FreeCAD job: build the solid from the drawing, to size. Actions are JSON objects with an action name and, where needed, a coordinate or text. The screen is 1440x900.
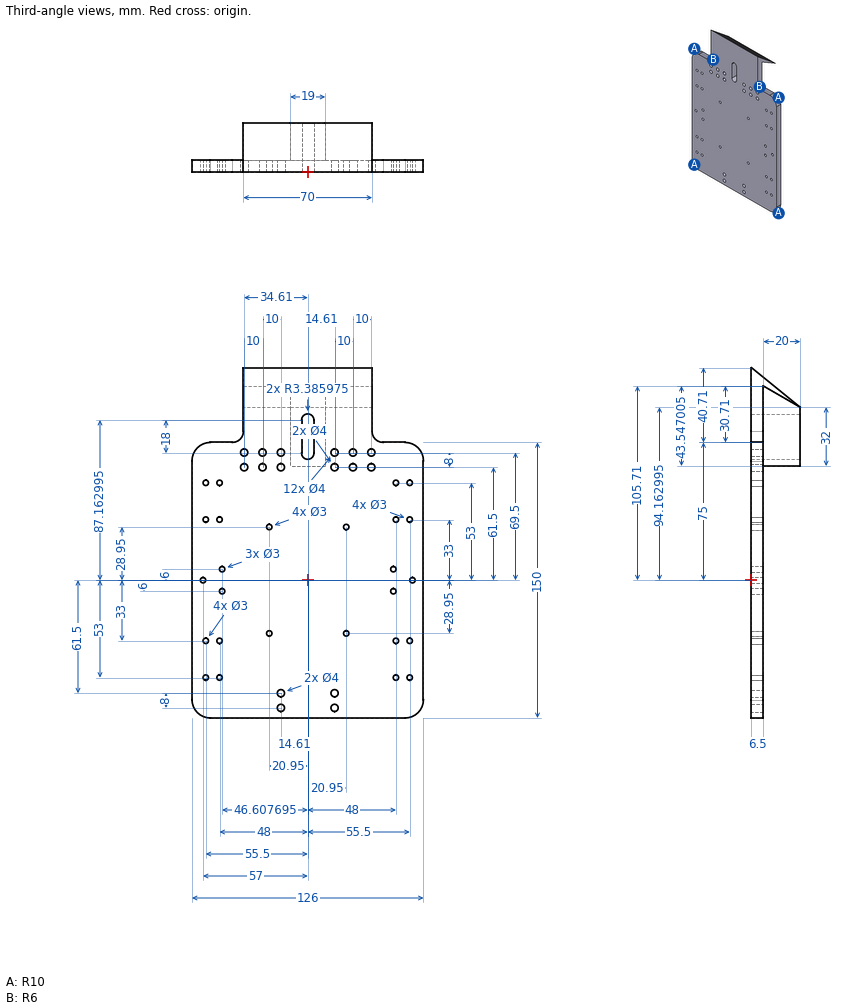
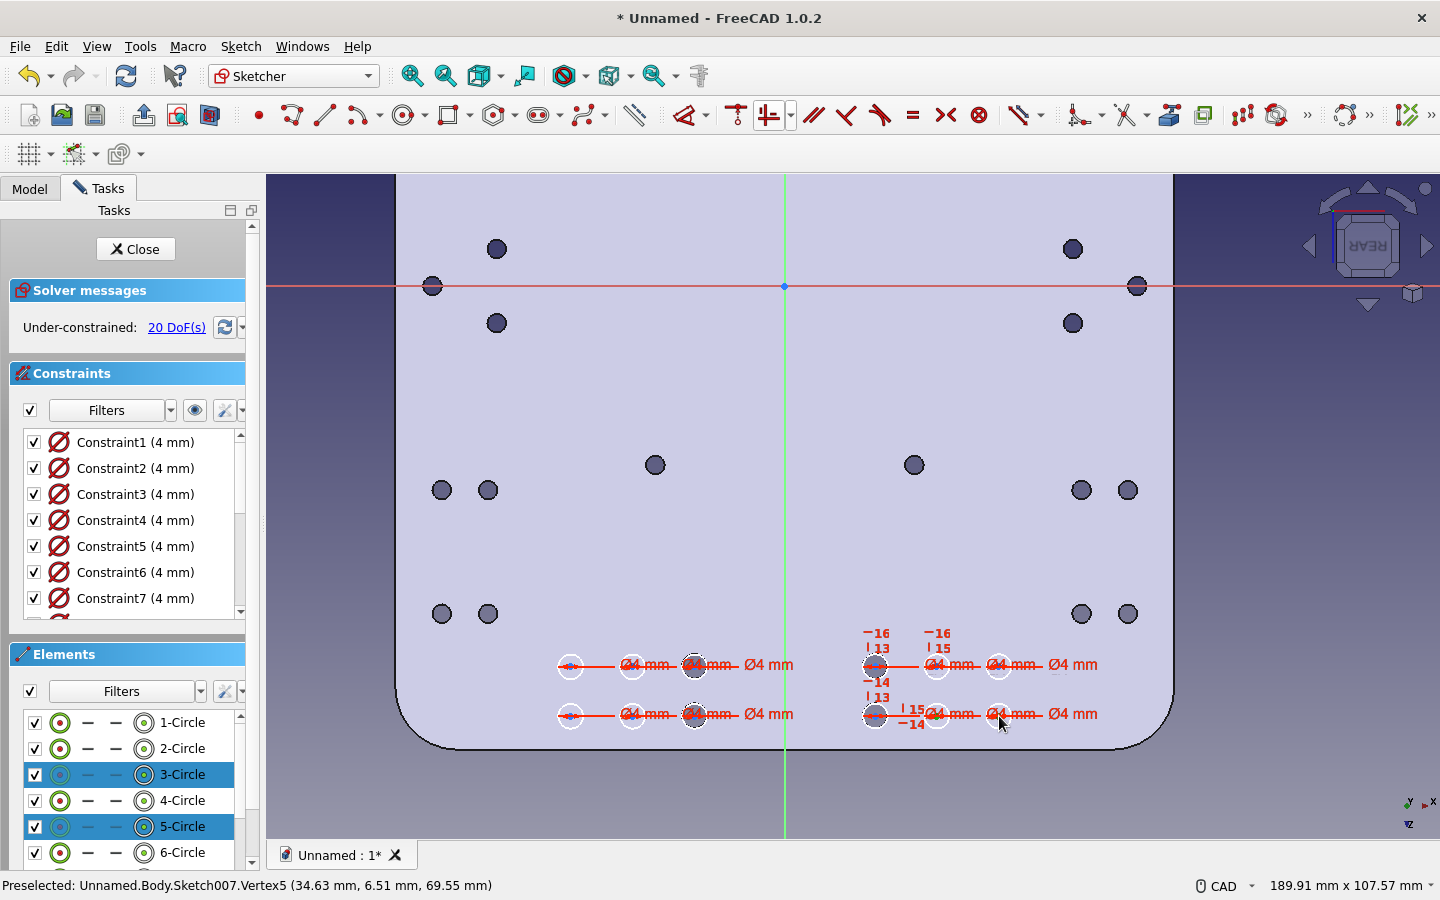
{"action": "left_click", "coordinate": [790, 116]}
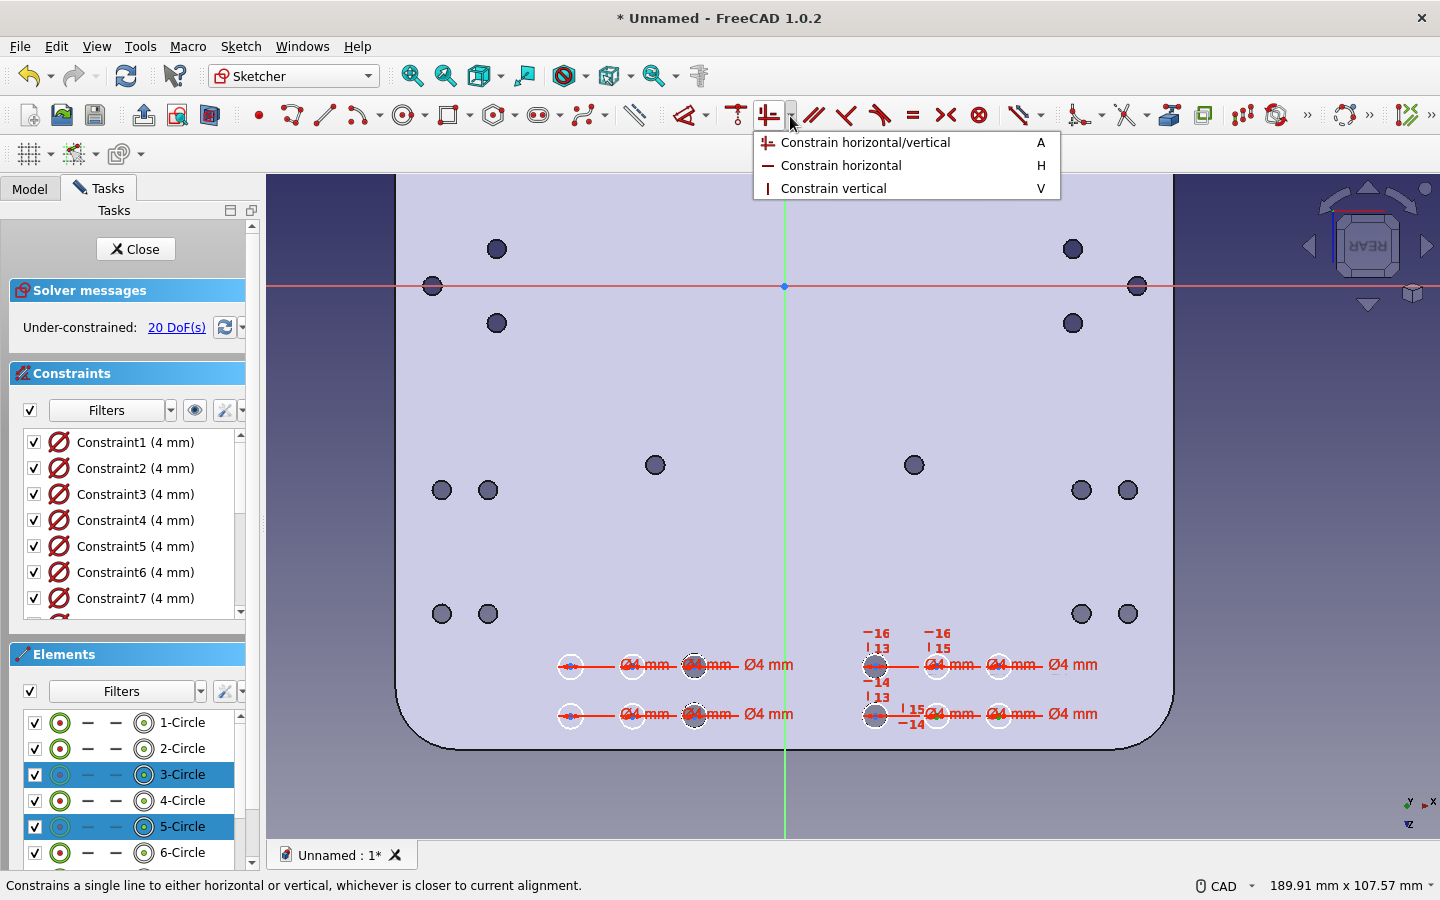
{"action": "left_click", "coordinate": [907, 166]}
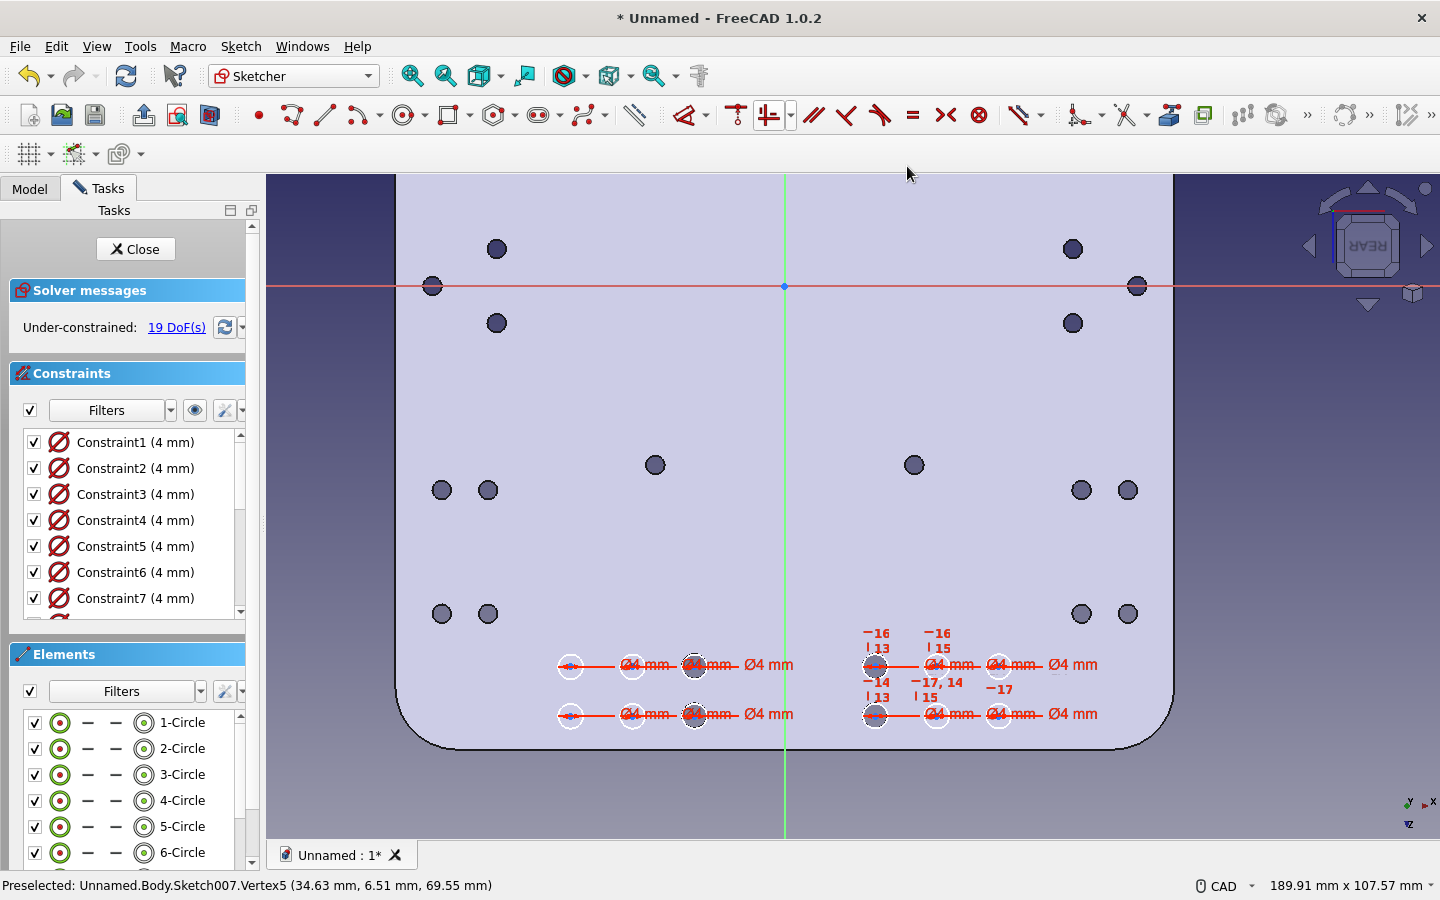
{"action": "left_click", "coordinate": [999, 716]}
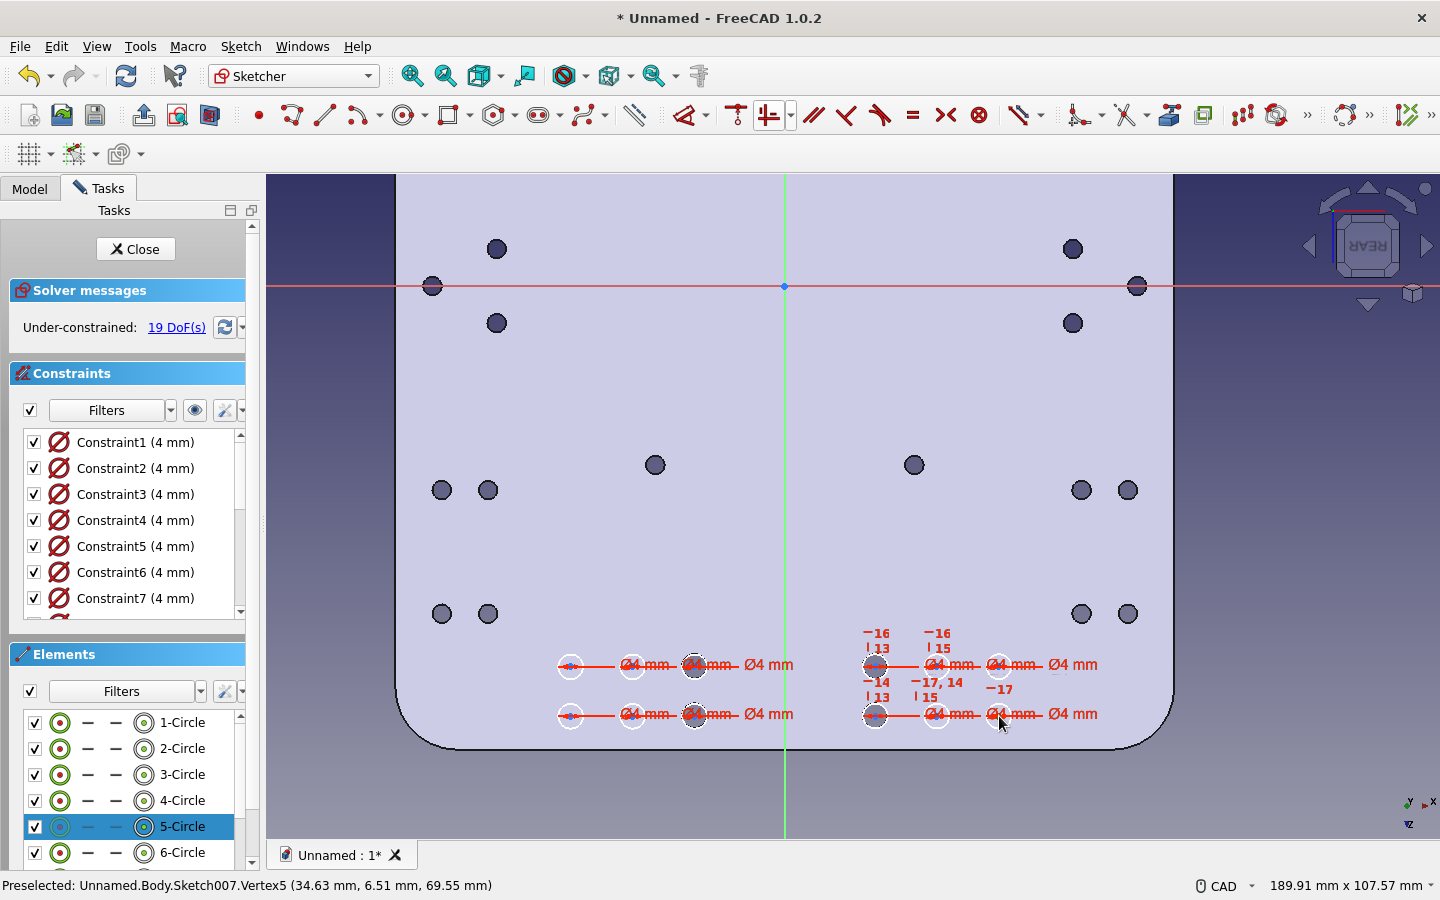
{"action": "left_click", "coordinate": [999, 667]}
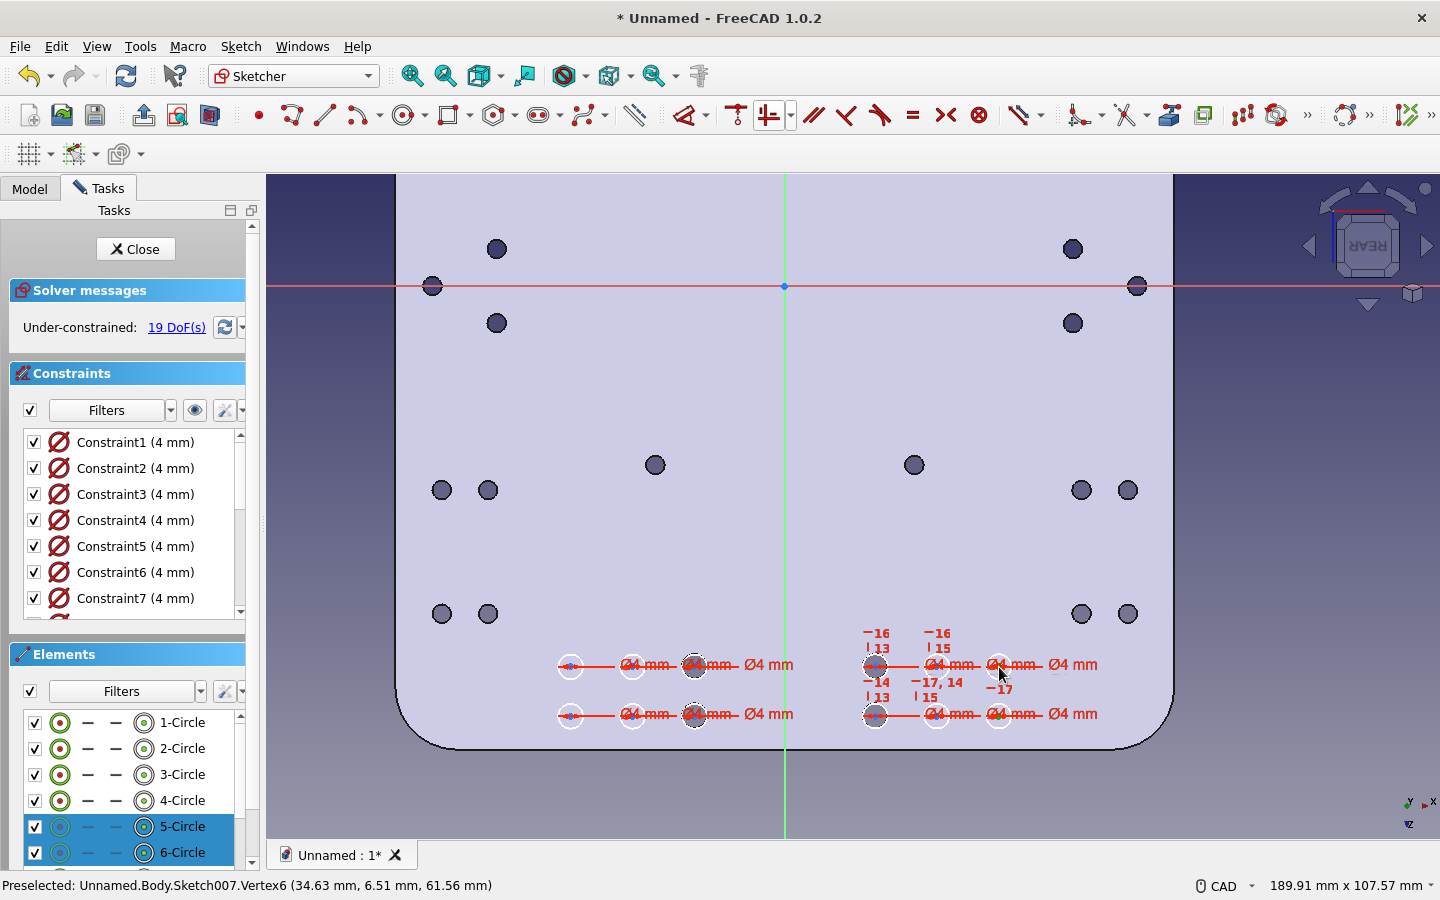
{"action": "key", "text": "v"}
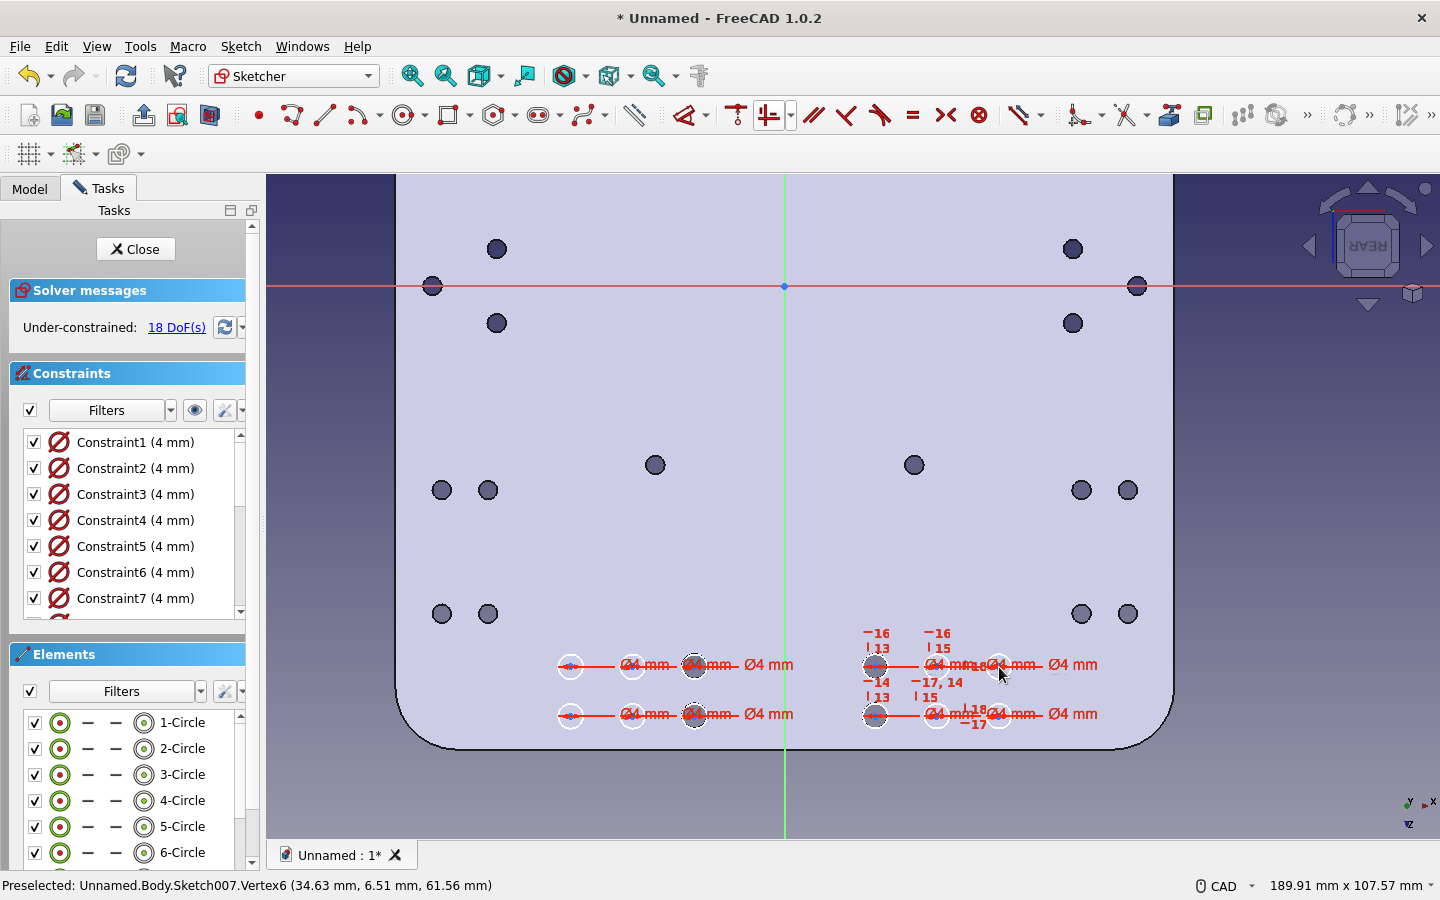
{"action": "left_click", "coordinate": [937, 667]}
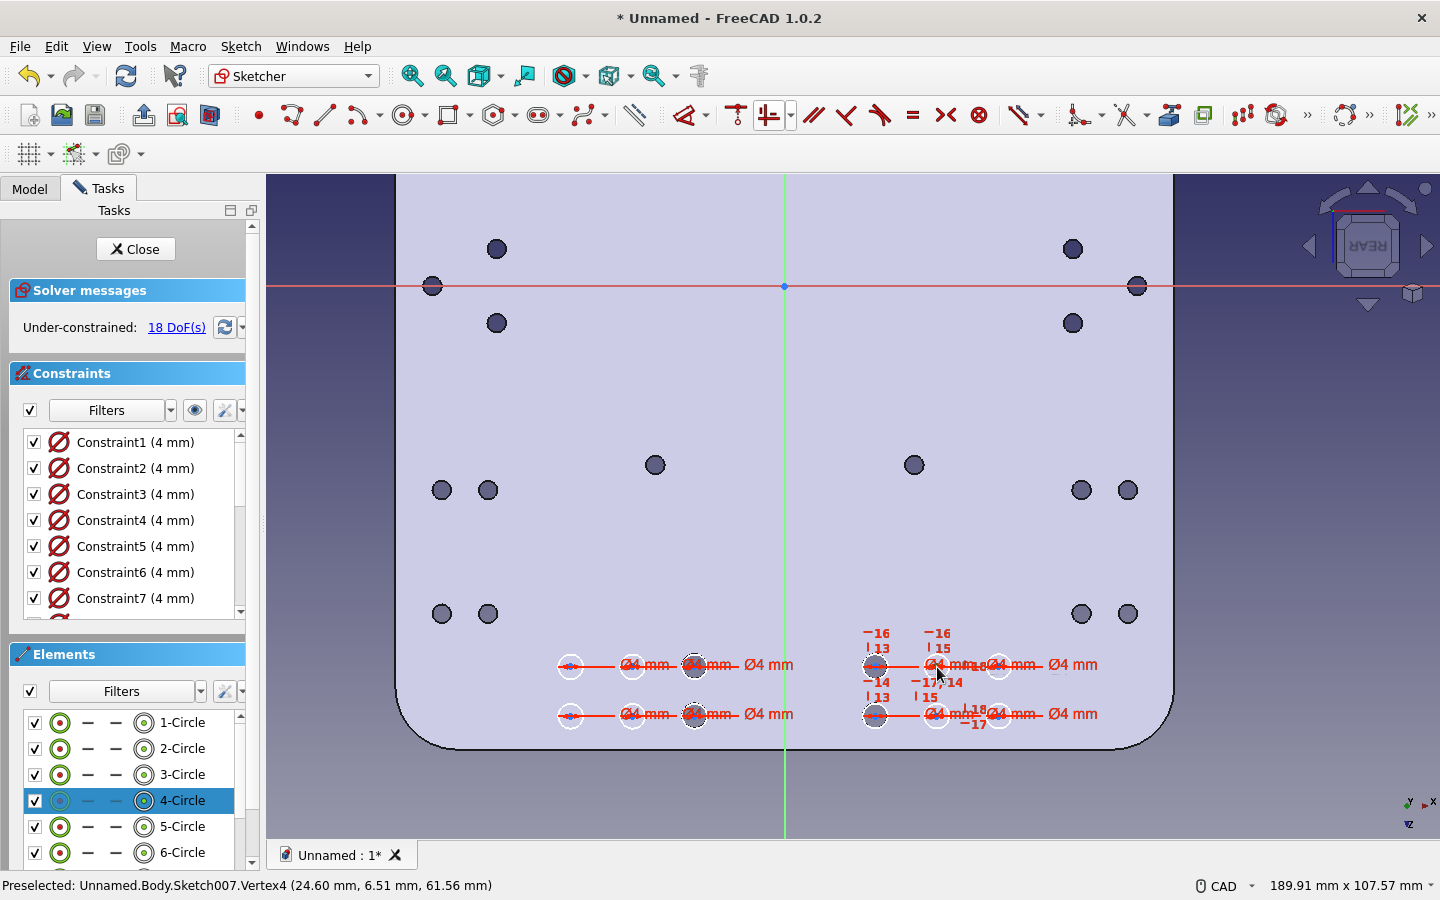
{"action": "left_click", "coordinate": [999, 667]}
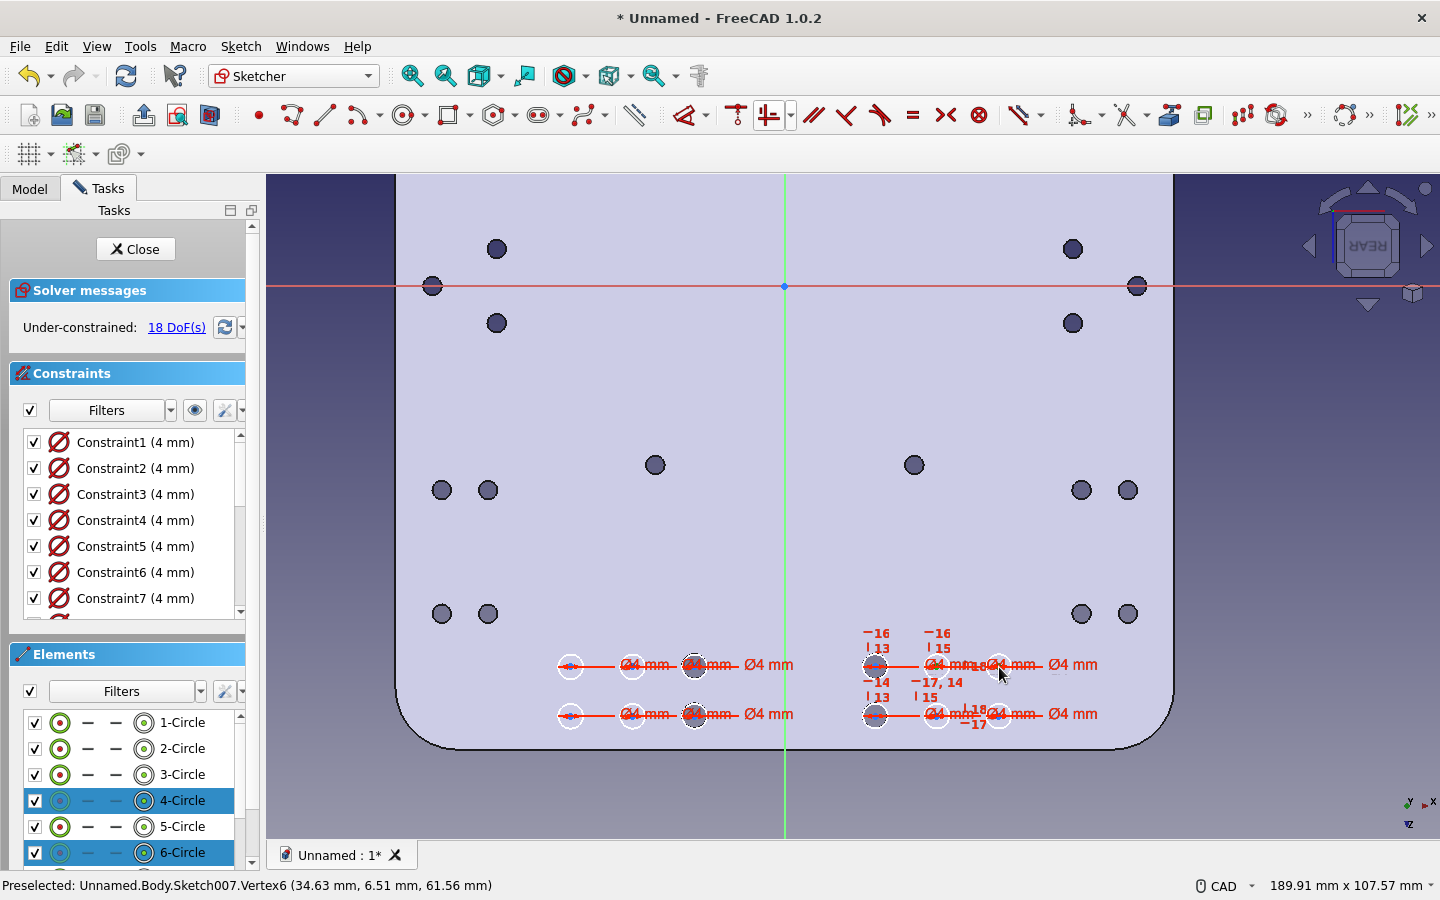
{"action": "key", "text": "h"}